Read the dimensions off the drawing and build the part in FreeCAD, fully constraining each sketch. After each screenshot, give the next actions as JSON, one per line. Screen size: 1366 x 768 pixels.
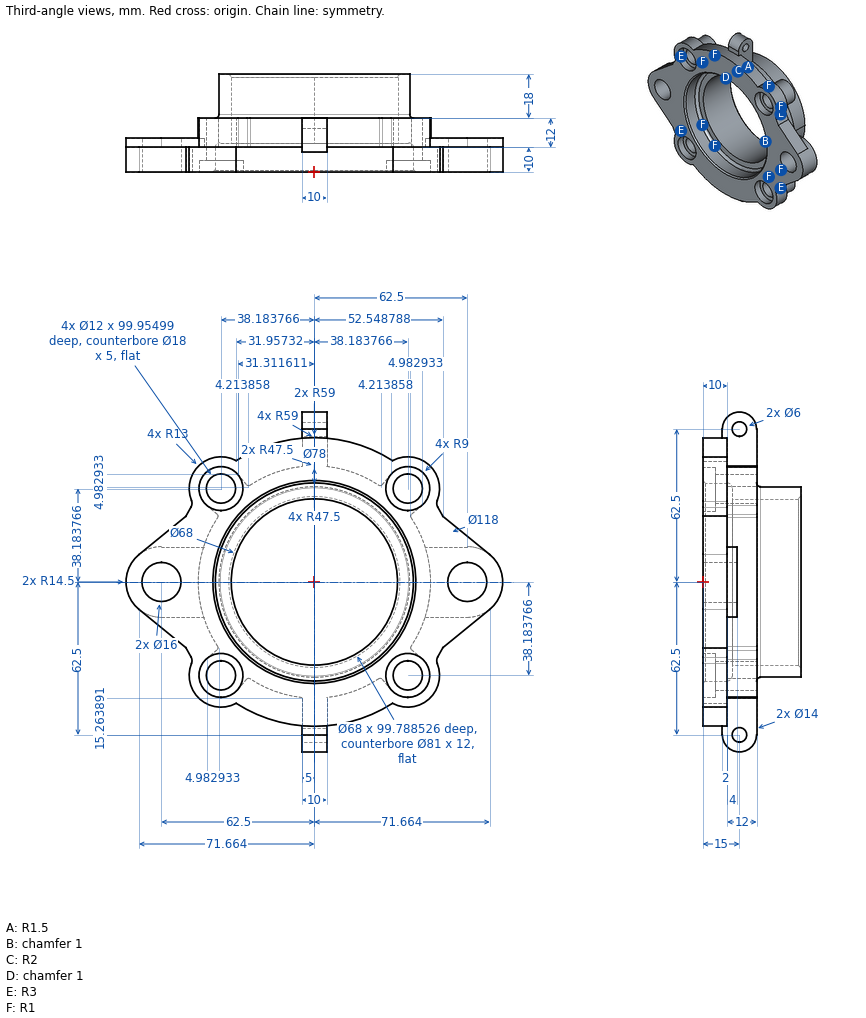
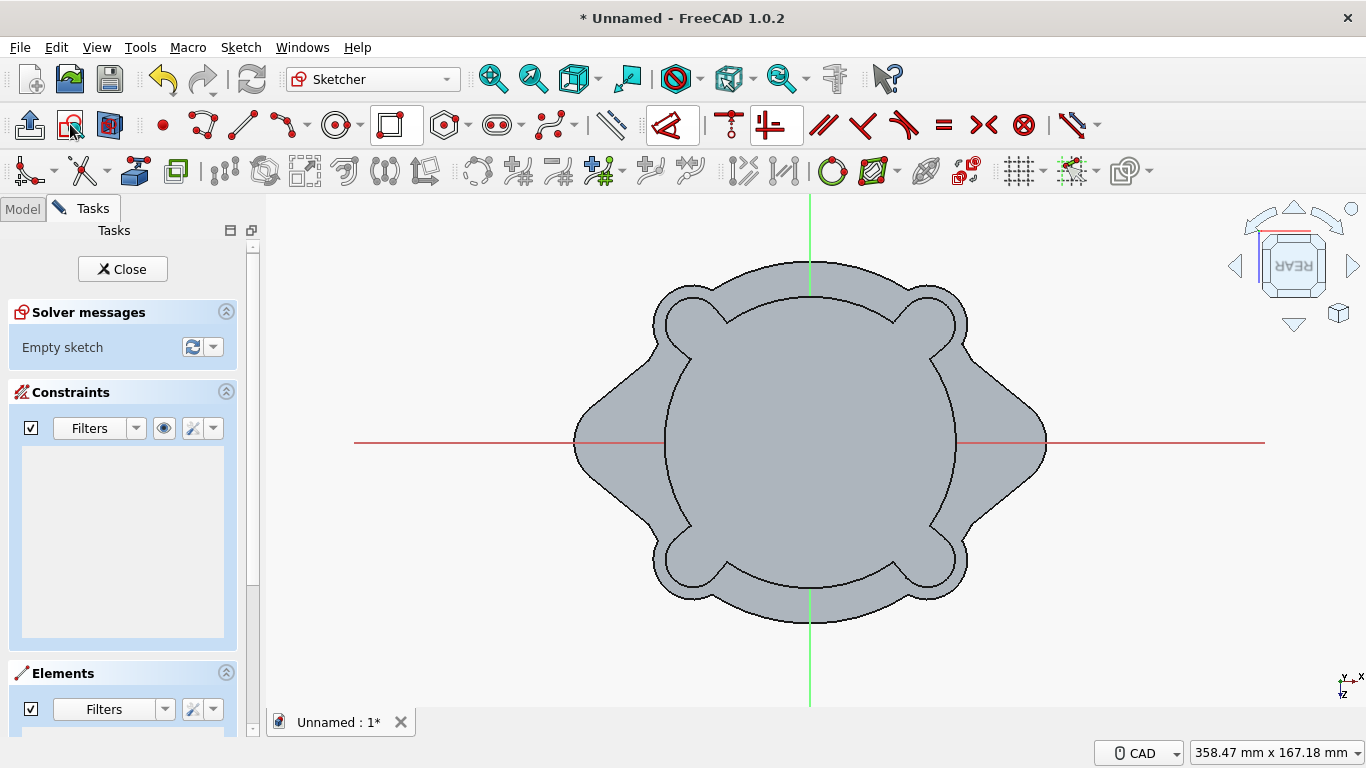
{"action": "left_click", "coordinate": [110, 126]}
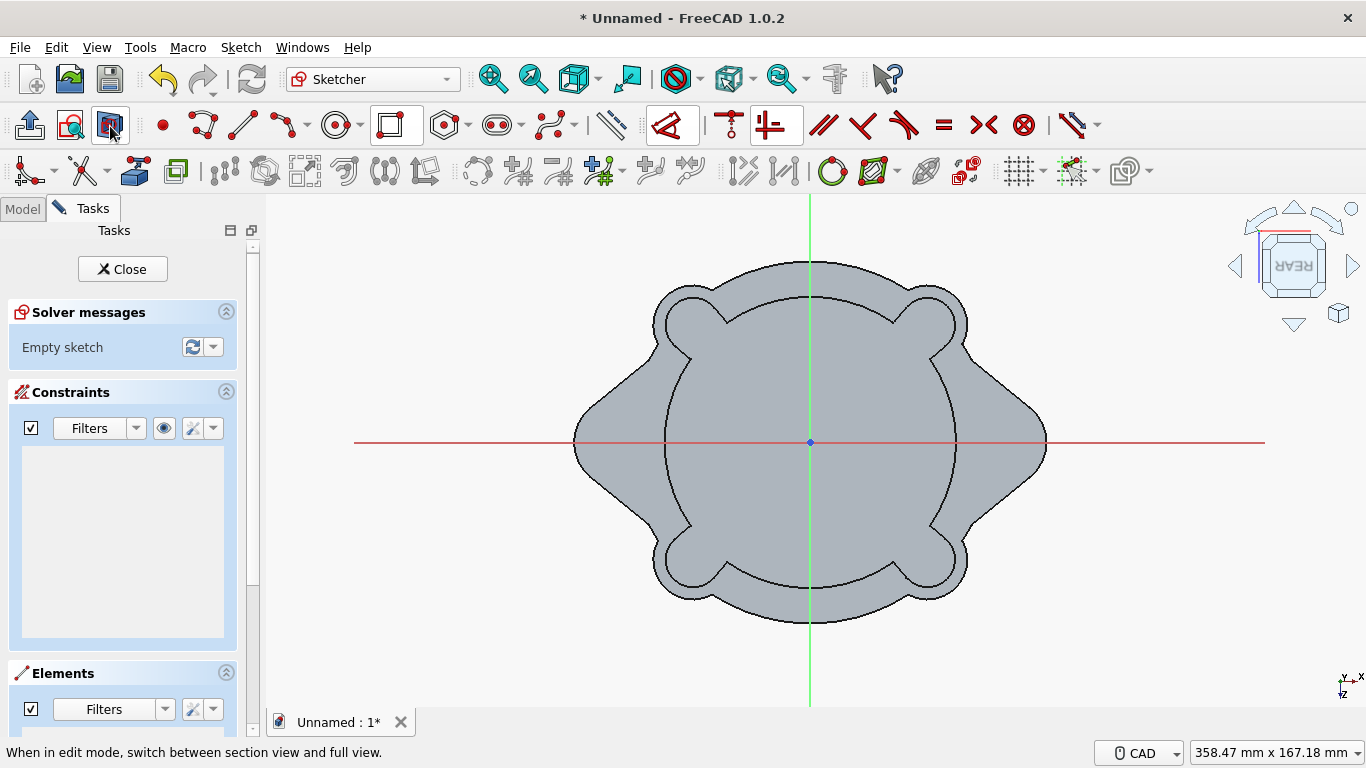
{"action": "left_click", "coordinate": [244, 126]}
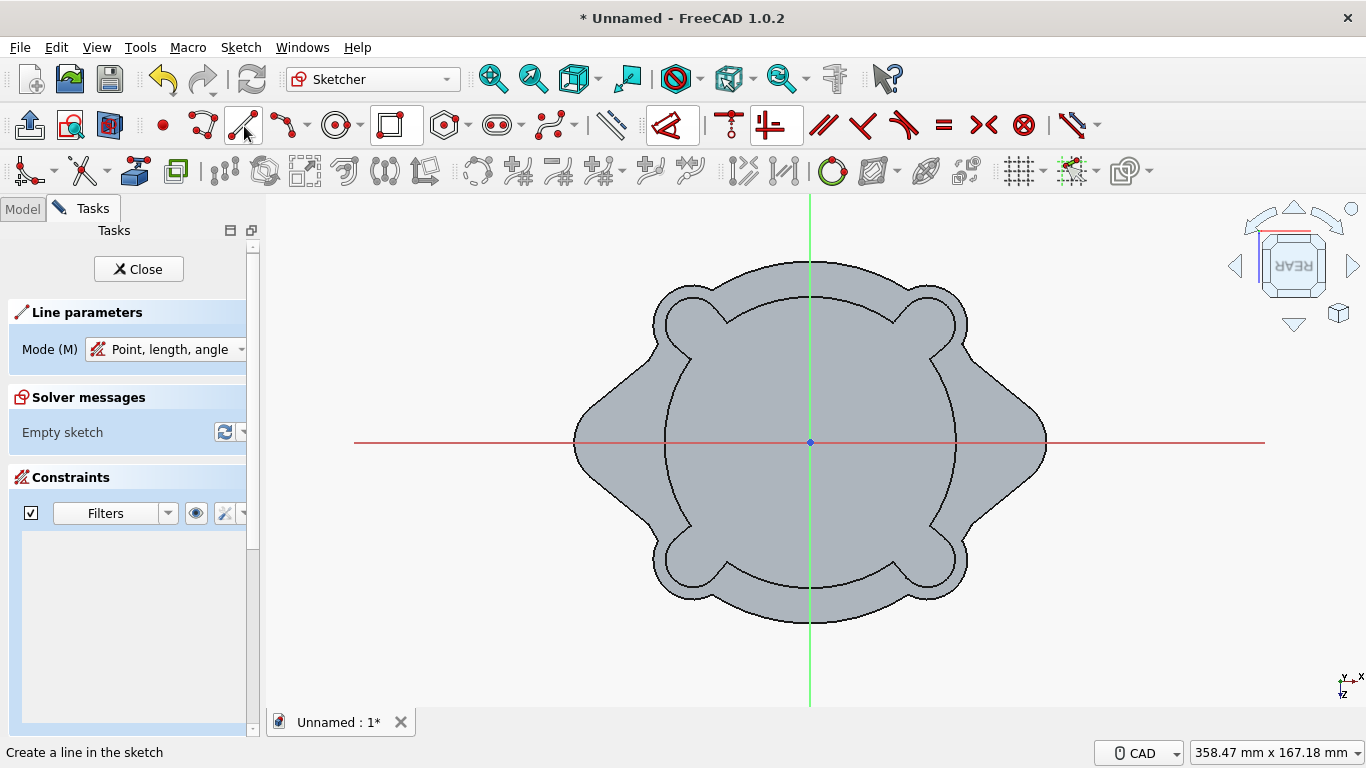
{"action": "left_click", "coordinate": [671, 398]}
{"action": "left_click", "coordinate": [619, 398]}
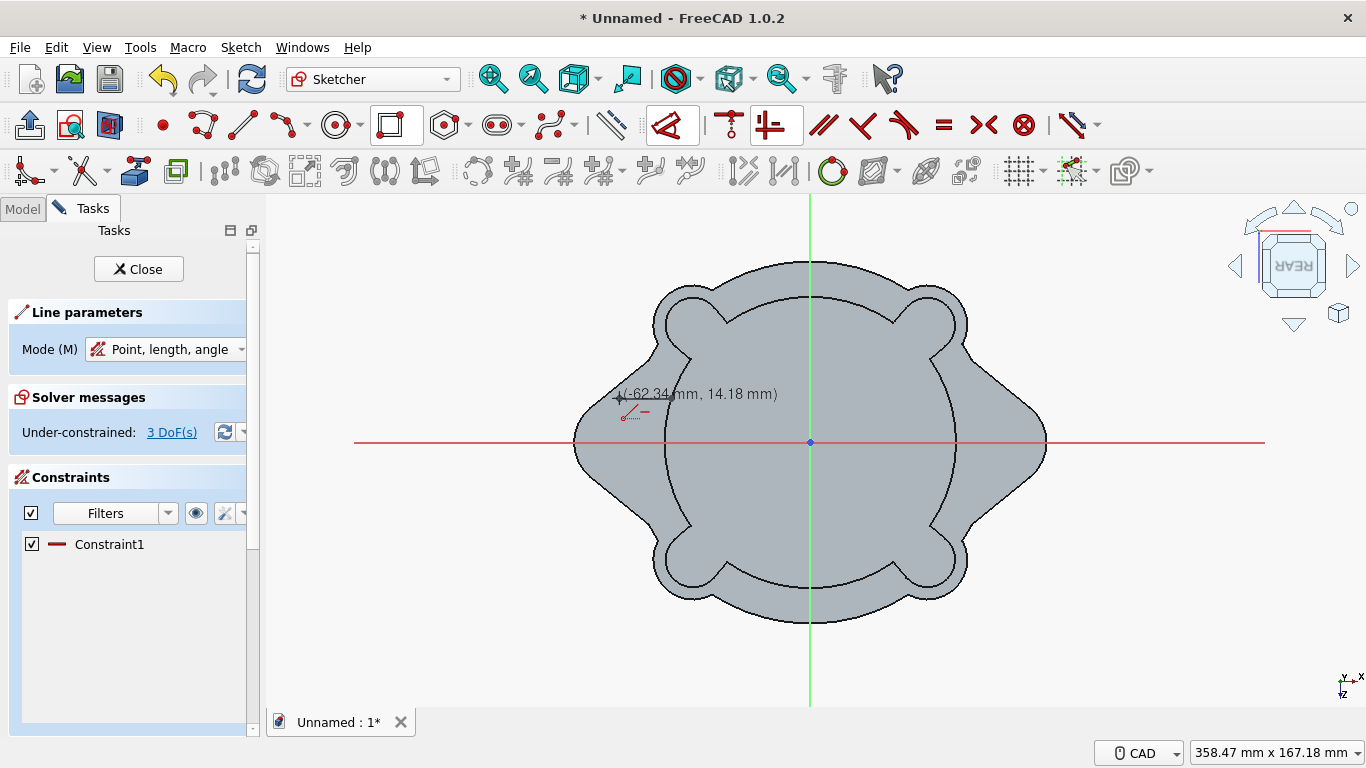
{"action": "left_click", "coordinate": [619, 487]}
{"action": "left_click", "coordinate": [671, 487]}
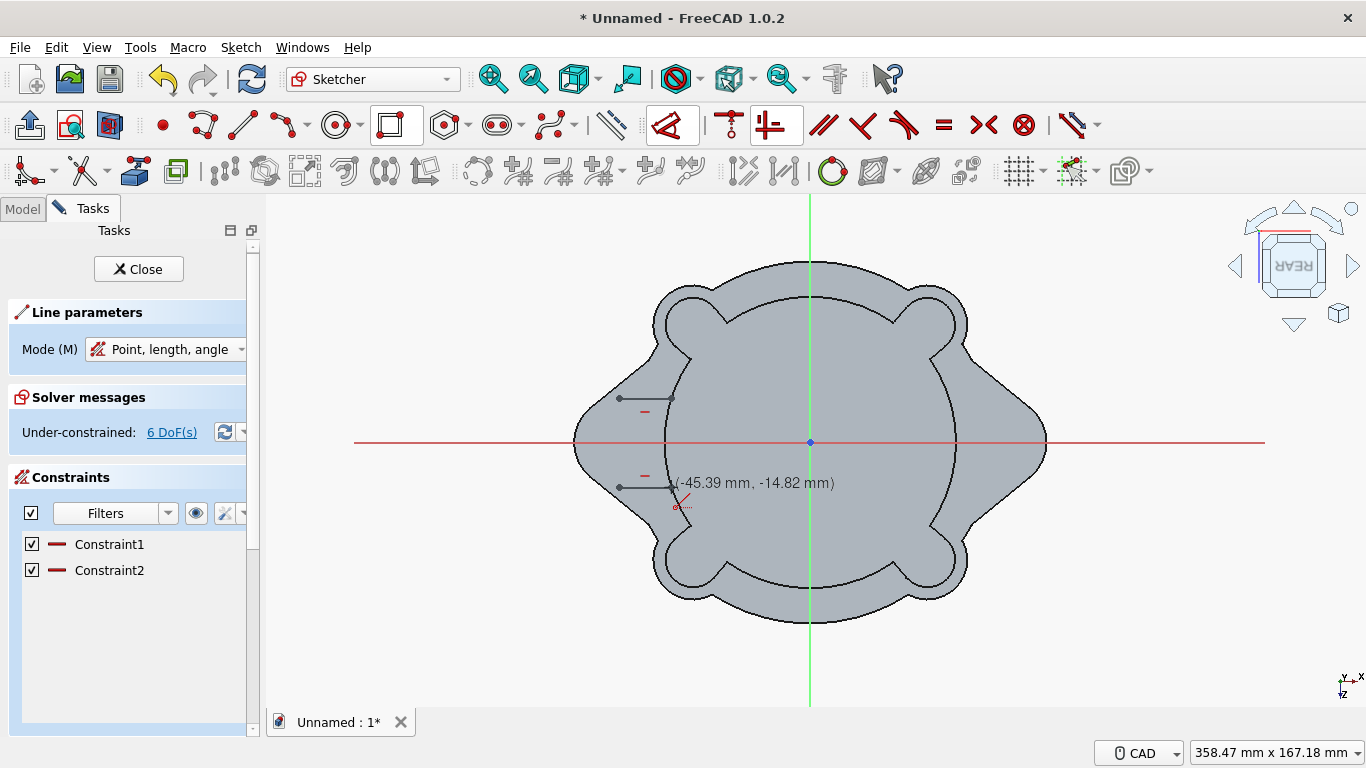
{"action": "left_click", "coordinate": [949, 487]}
{"action": "left_click", "coordinate": [1002, 487]}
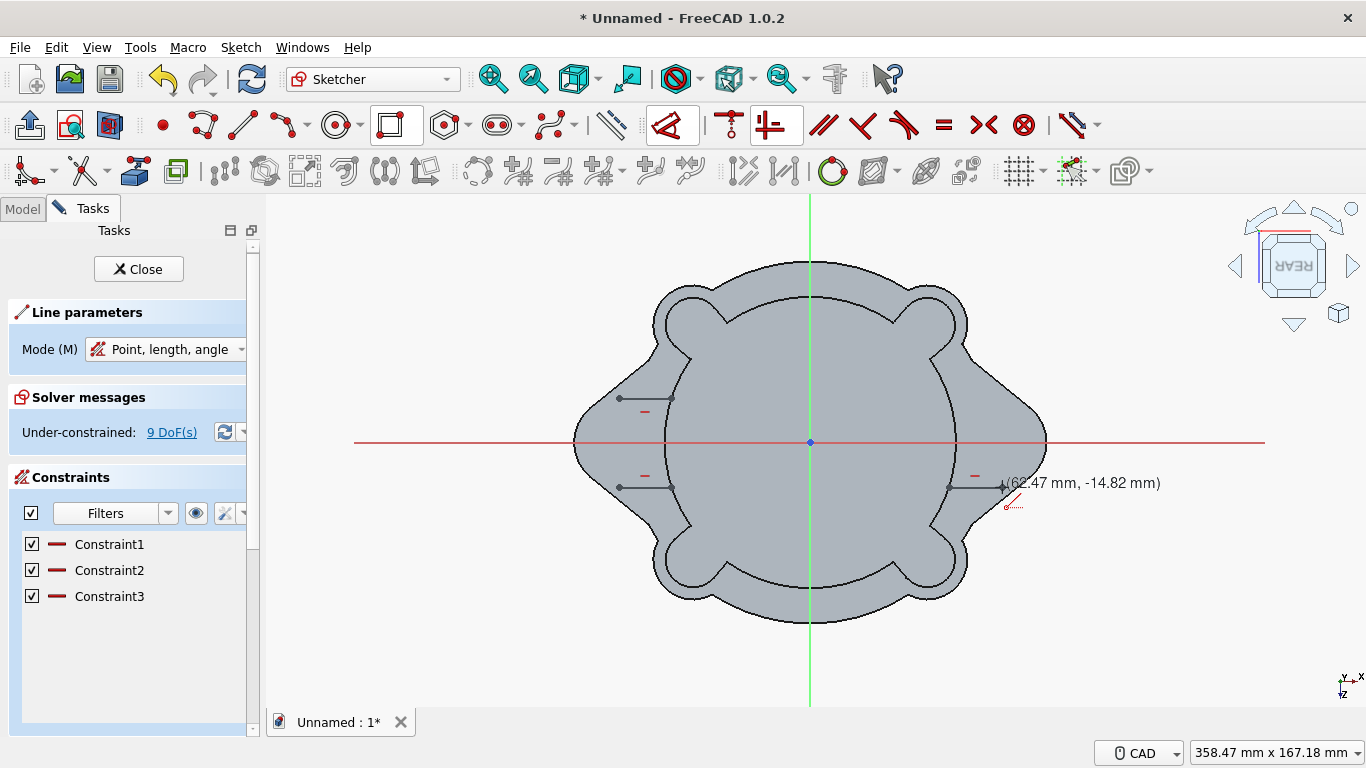
{"action": "left_click", "coordinate": [1002, 398]}
{"action": "left_click", "coordinate": [949, 398]}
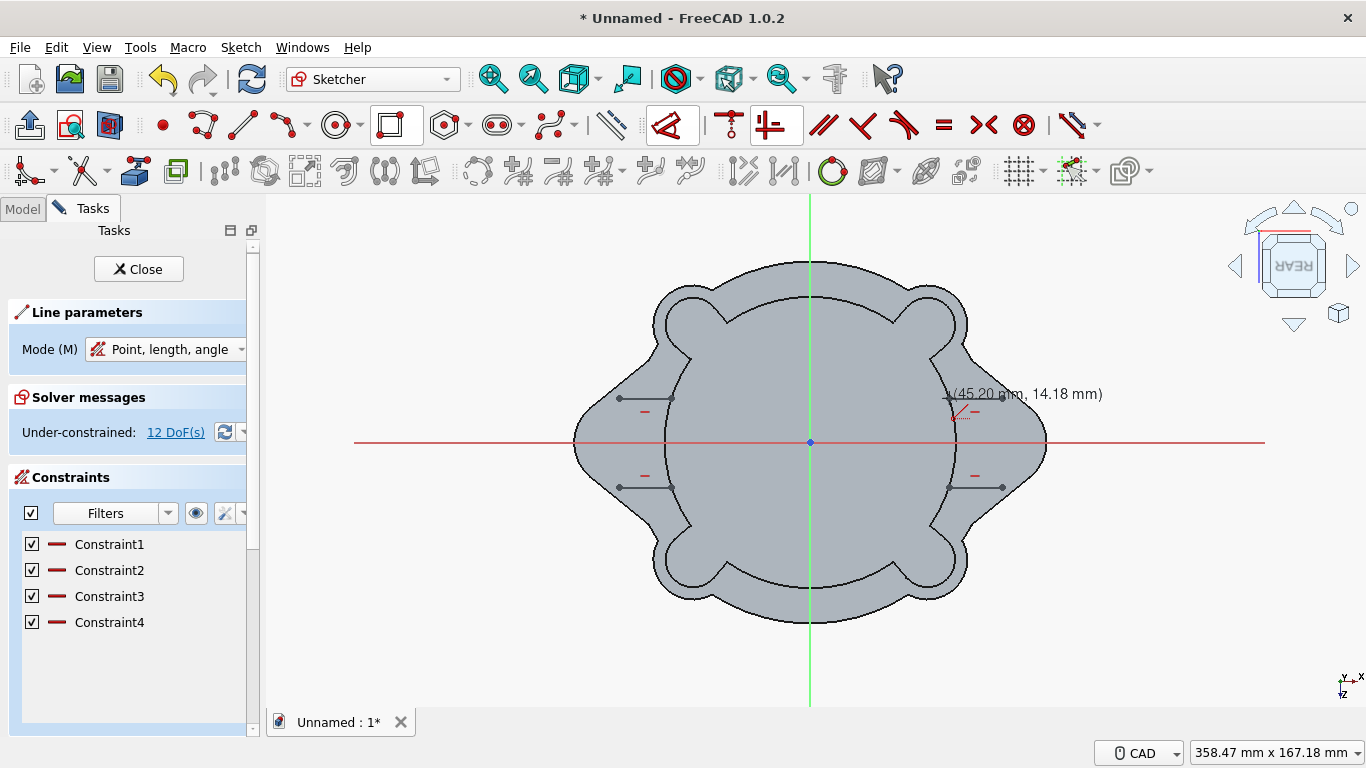
{"action": "left_click", "coordinate": [284, 126]}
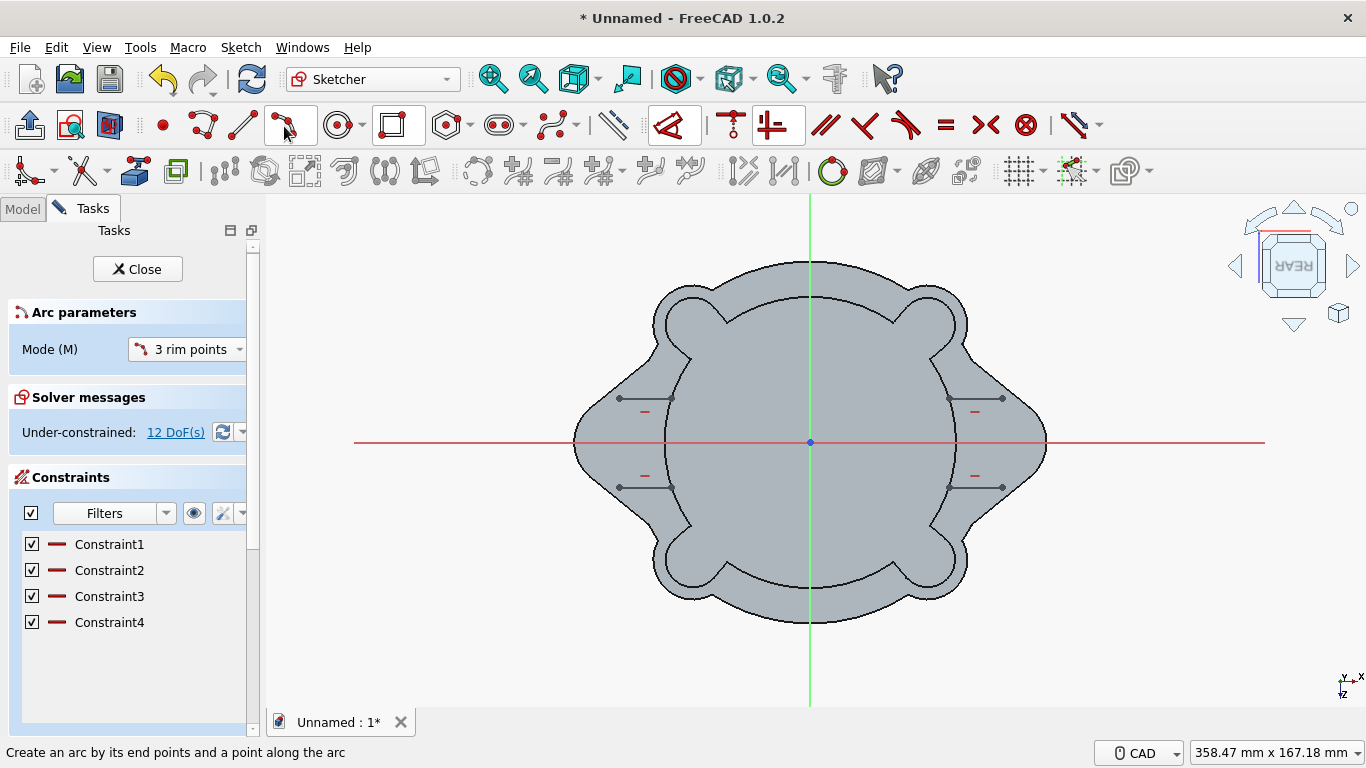
{"action": "left_click", "coordinate": [619, 399]}
{"action": "left_click", "coordinate": [619, 488]}
{"action": "left_click", "coordinate": [583, 416]}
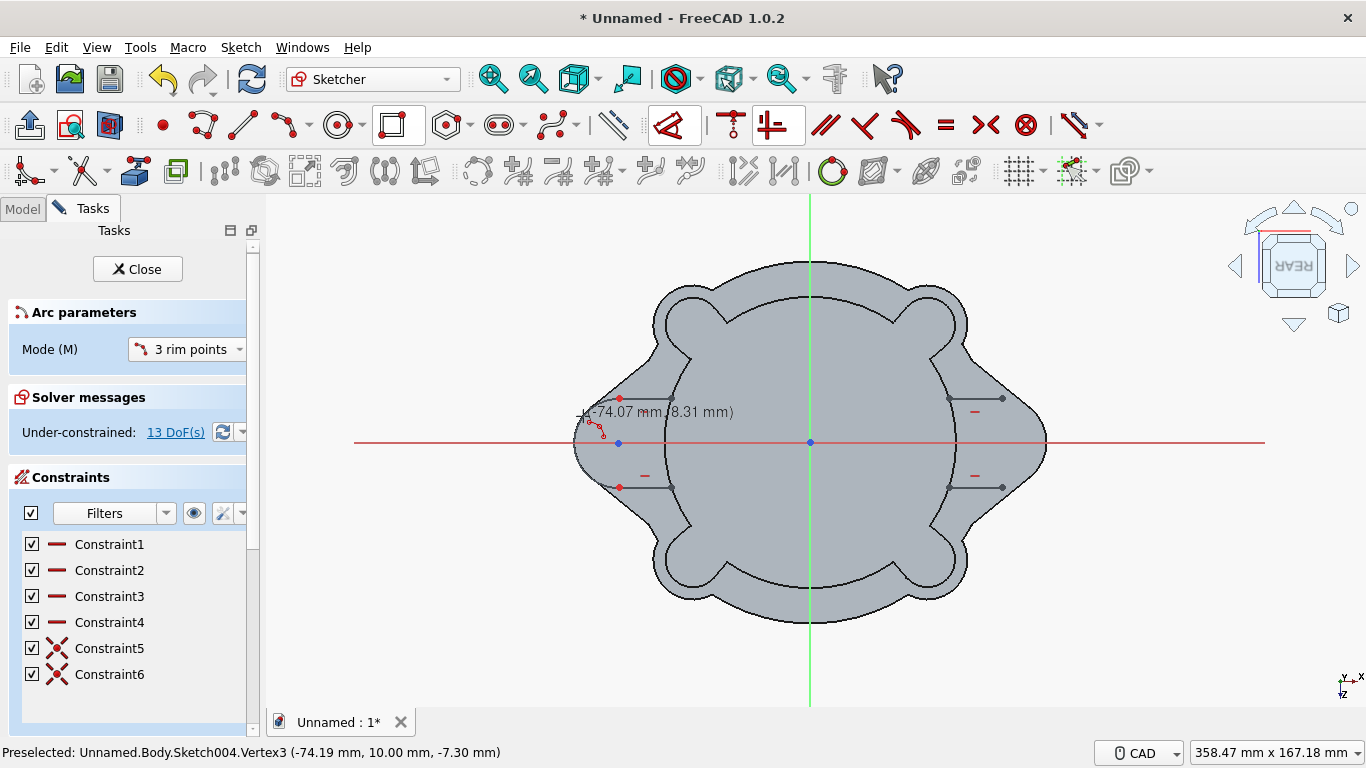
{"action": "left_click", "coordinate": [671, 488]}
{"action": "left_click", "coordinate": [949, 488]}
{"action": "left_click", "coordinate": [774, 584]}